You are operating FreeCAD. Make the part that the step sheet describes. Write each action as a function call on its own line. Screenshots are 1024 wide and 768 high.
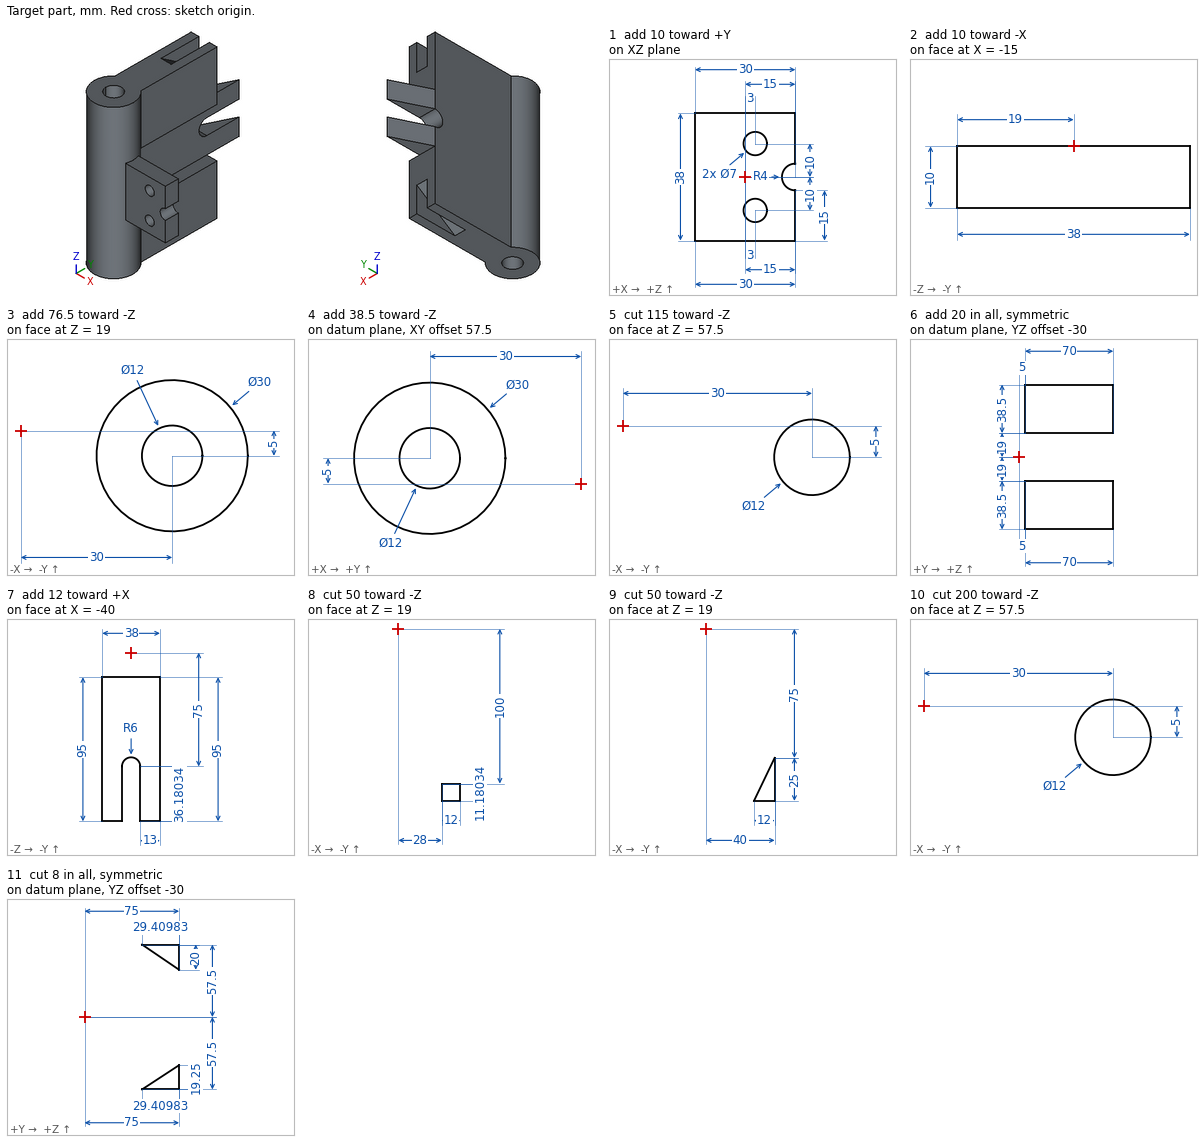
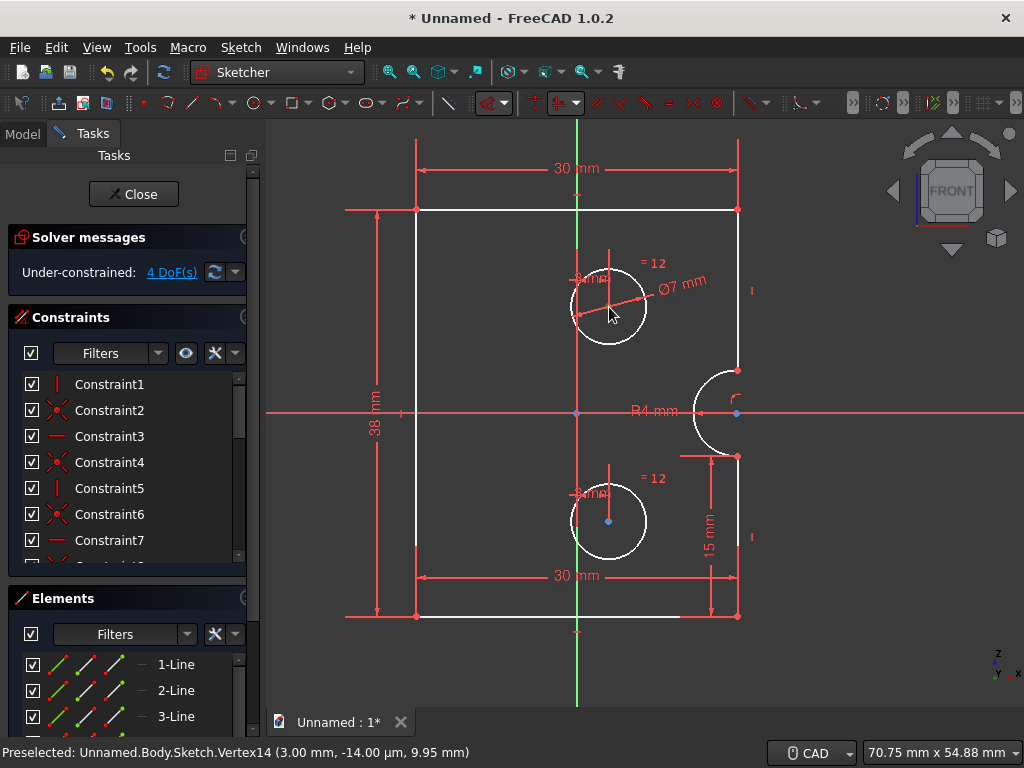
click(506, 104)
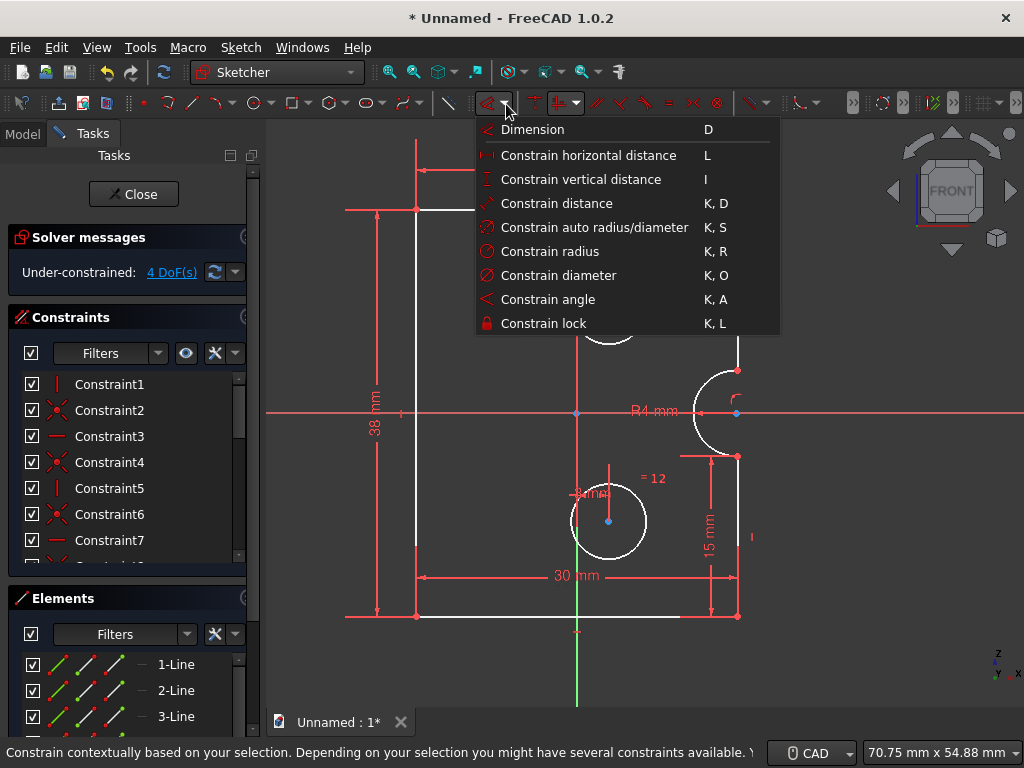
click(628, 179)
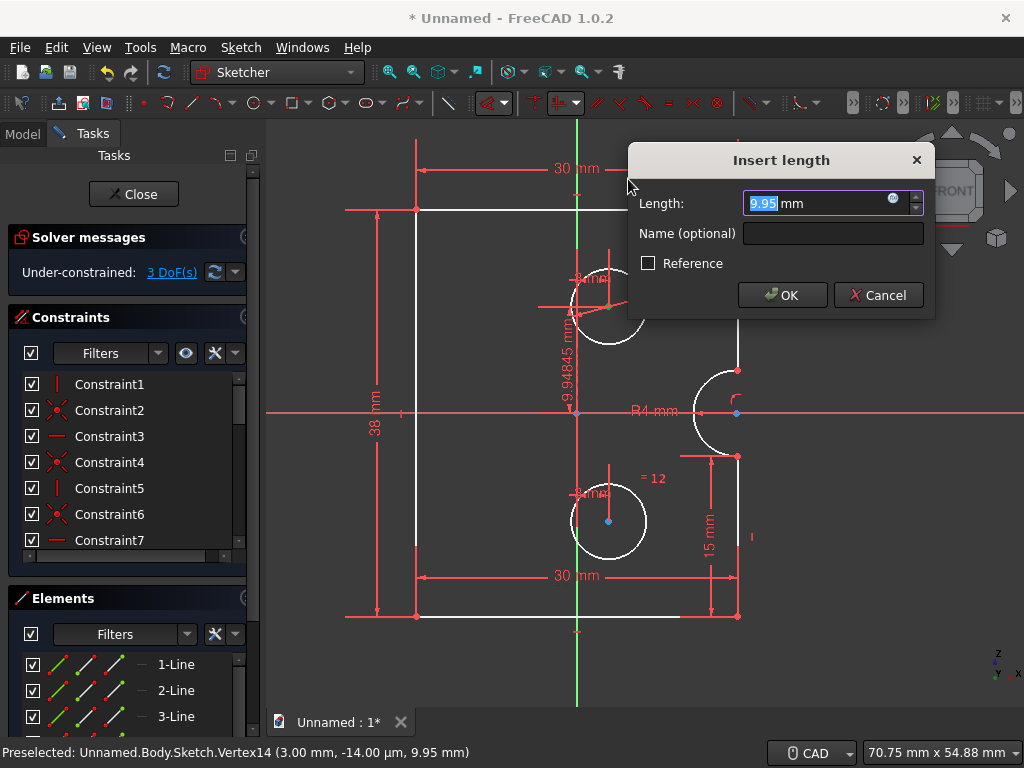
text(10)
key(Return)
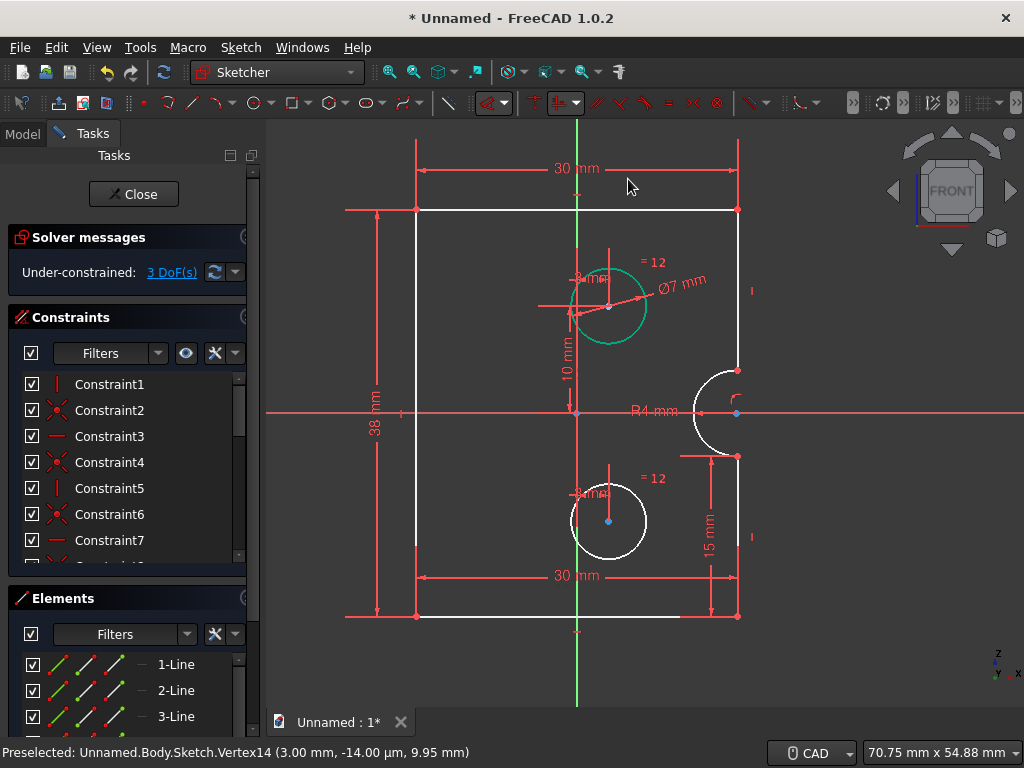
click(609, 522)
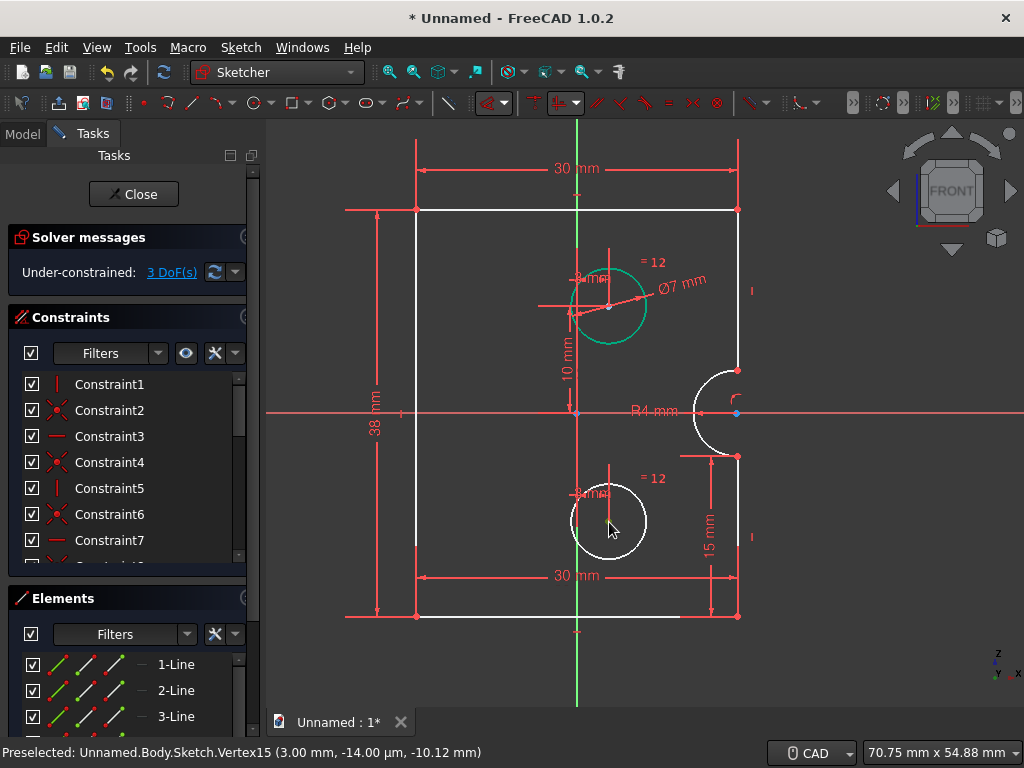
click(506, 104)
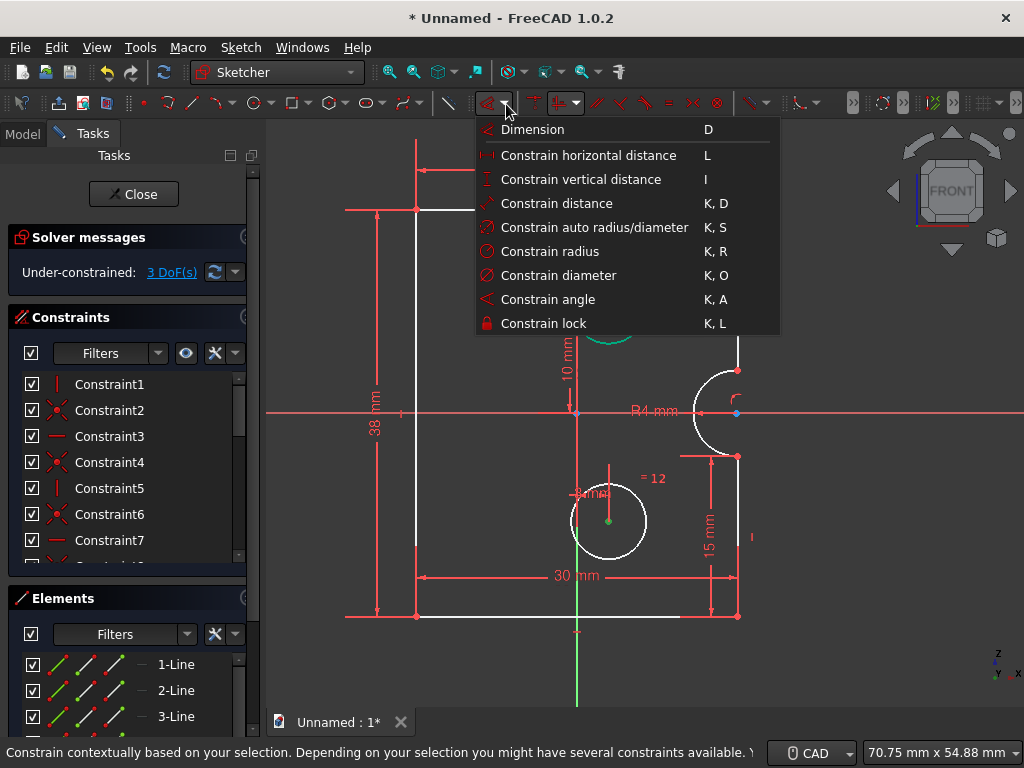
click(628, 179)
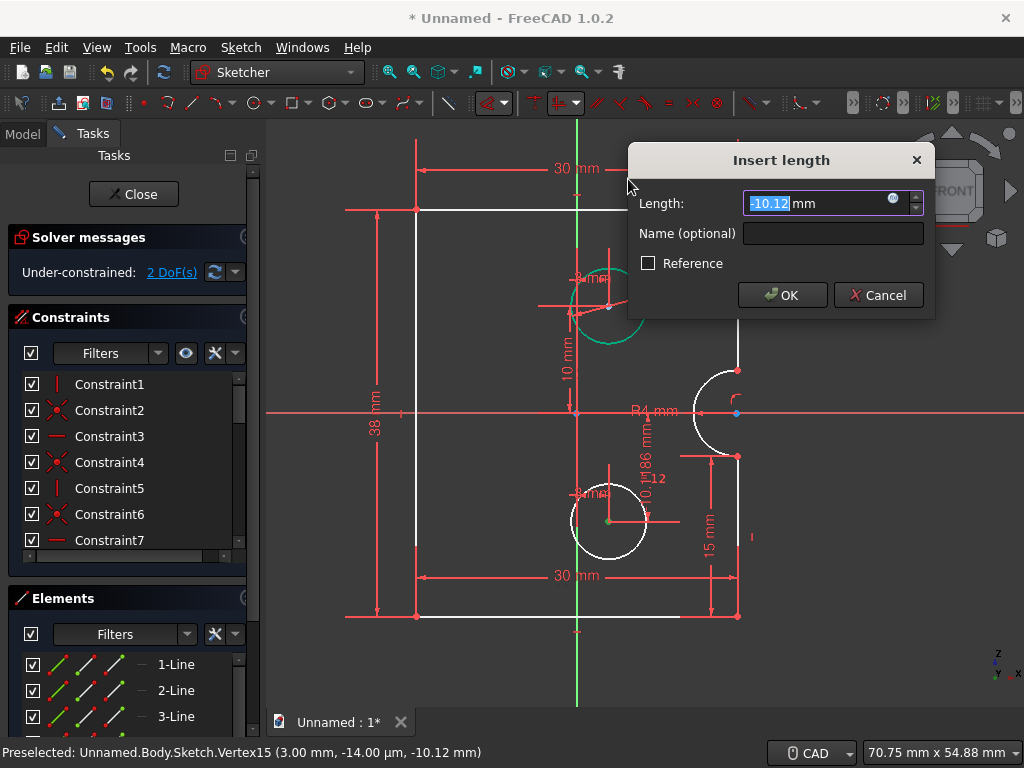
text(-10)
key(Return)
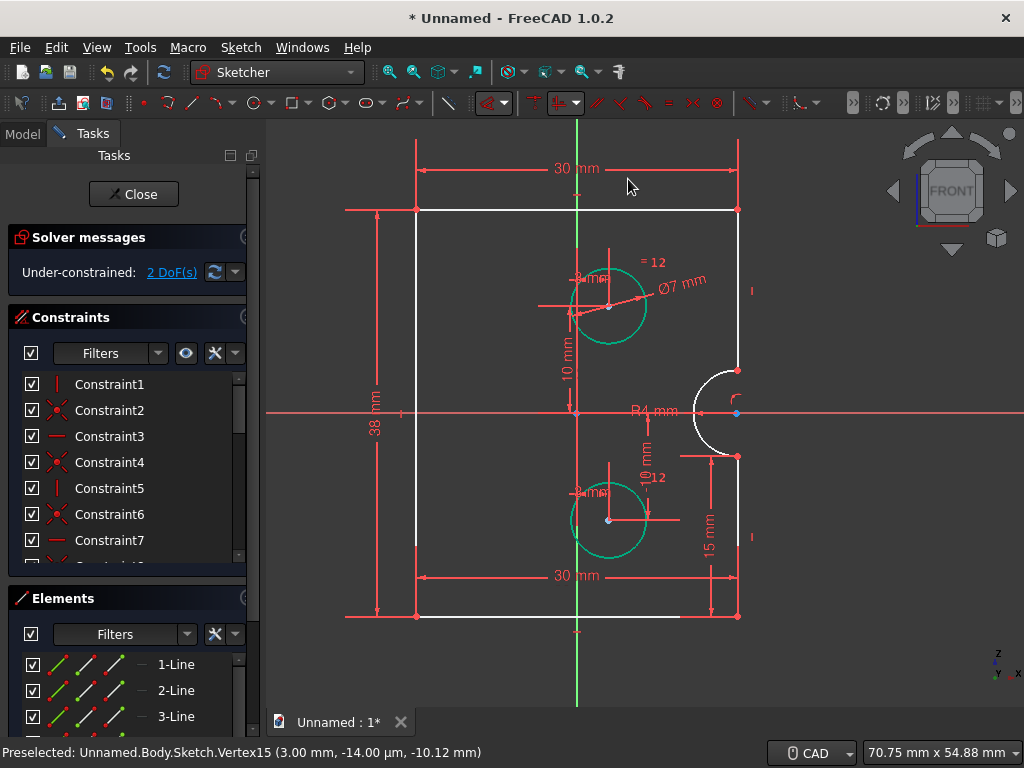
click(738, 456)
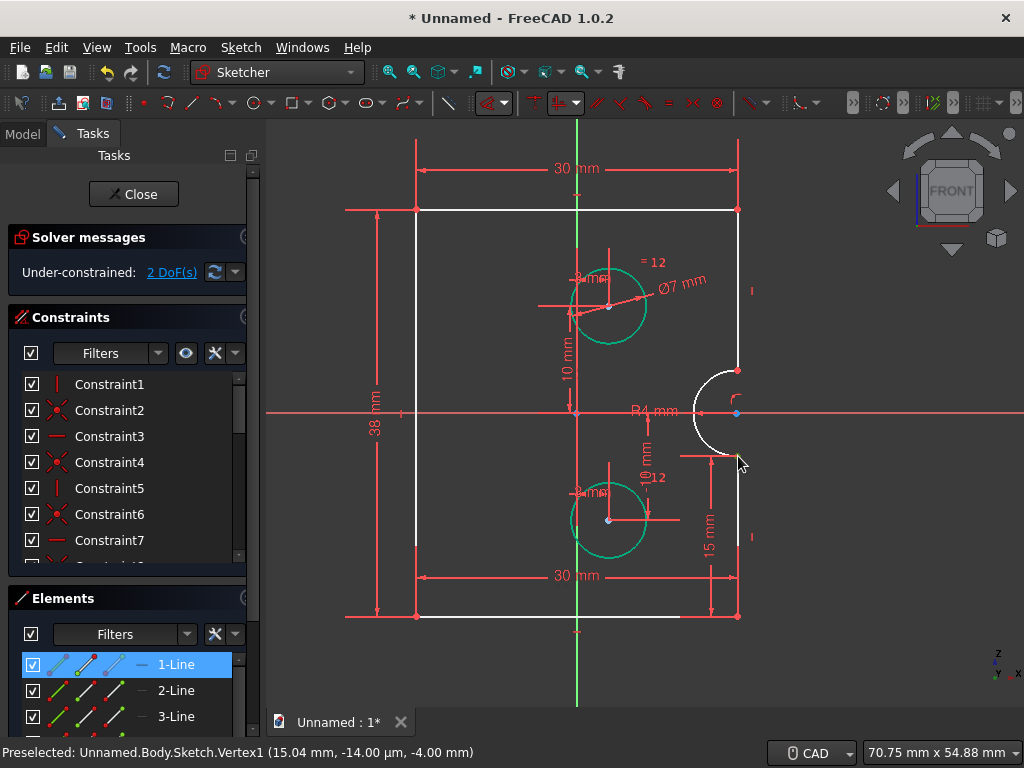
key(l)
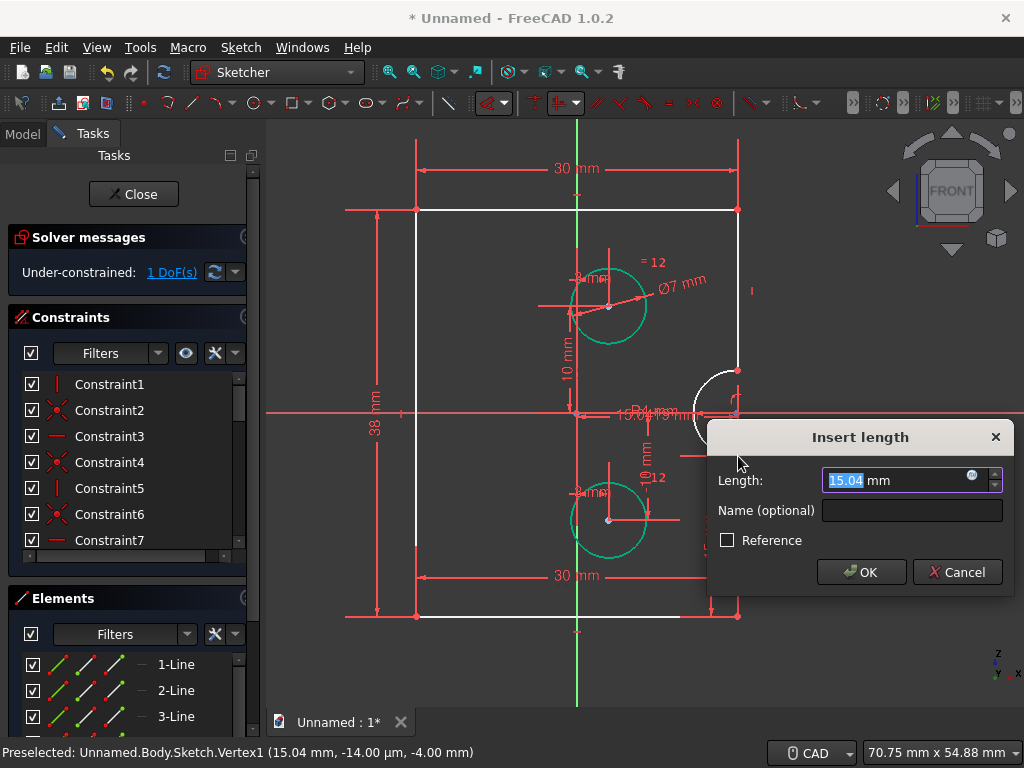
text(15)
key(Return)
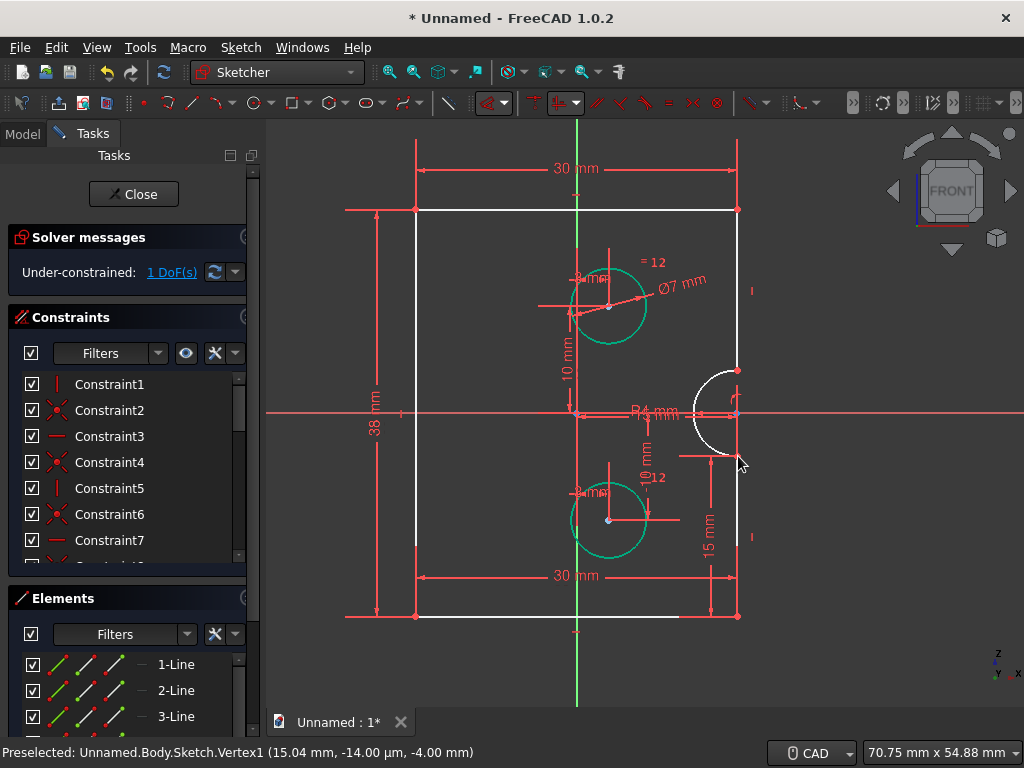
click(736, 413)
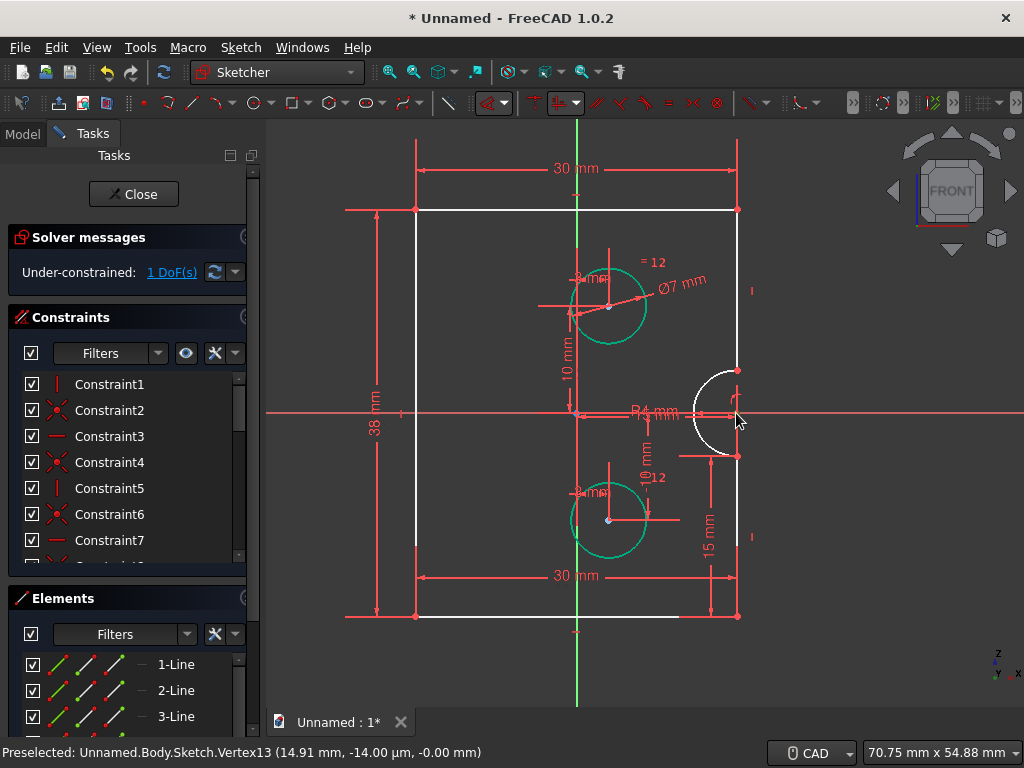
click(506, 104)